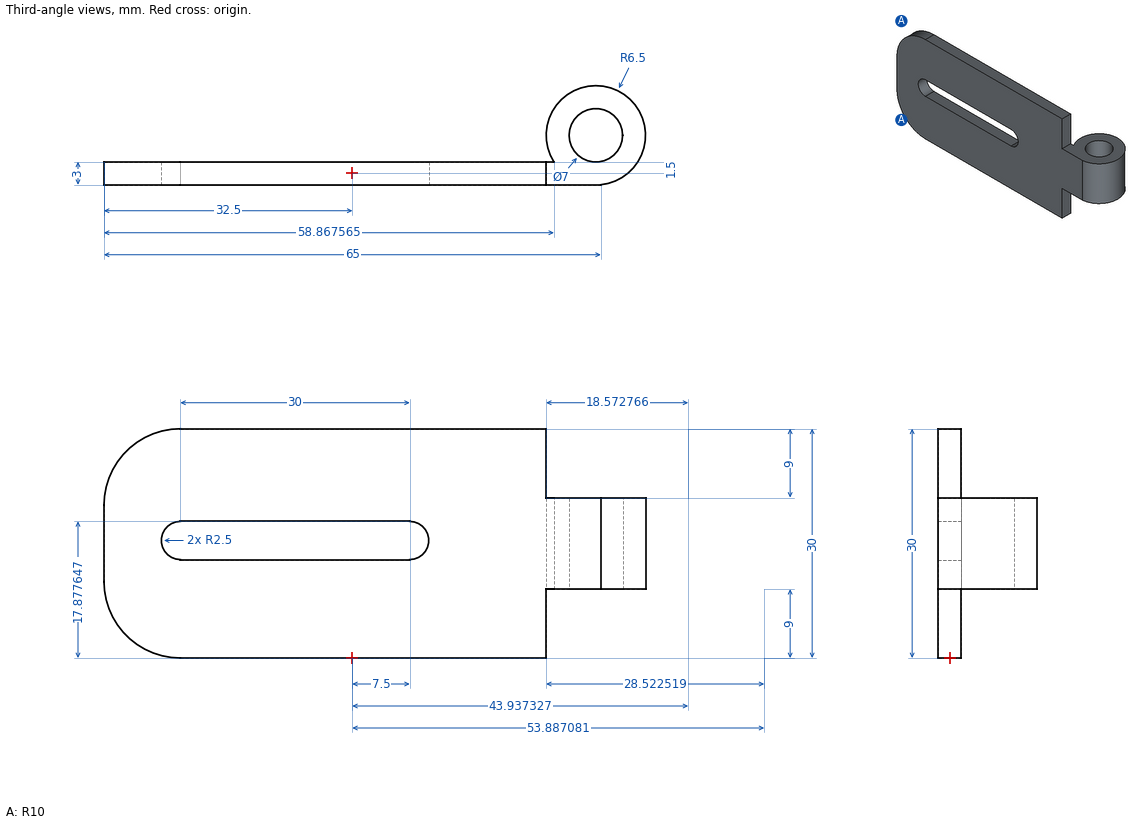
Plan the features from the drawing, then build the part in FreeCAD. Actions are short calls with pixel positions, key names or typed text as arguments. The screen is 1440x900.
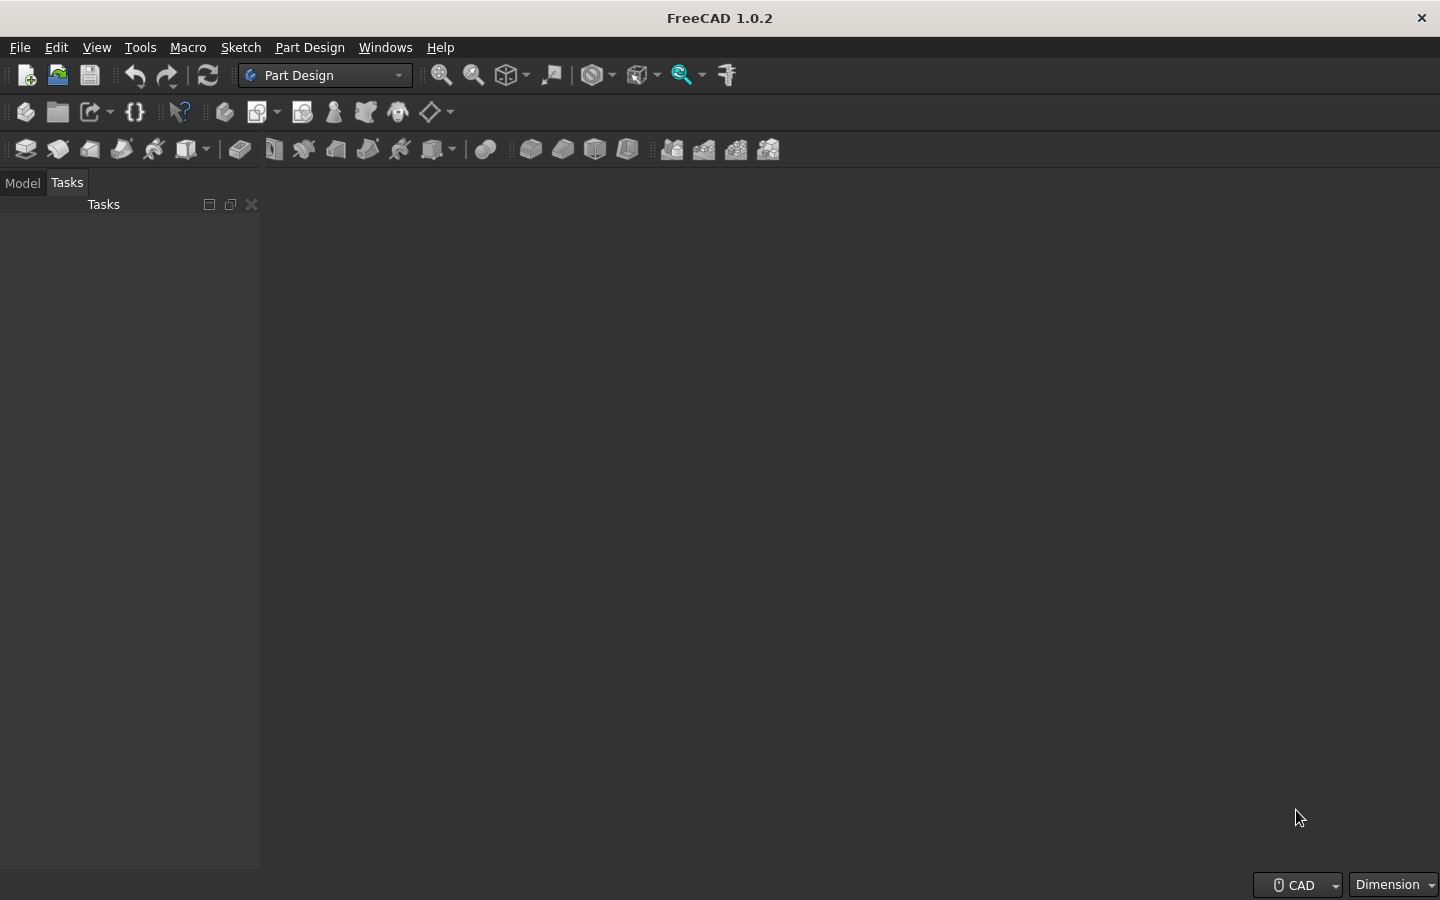
click(286, 112)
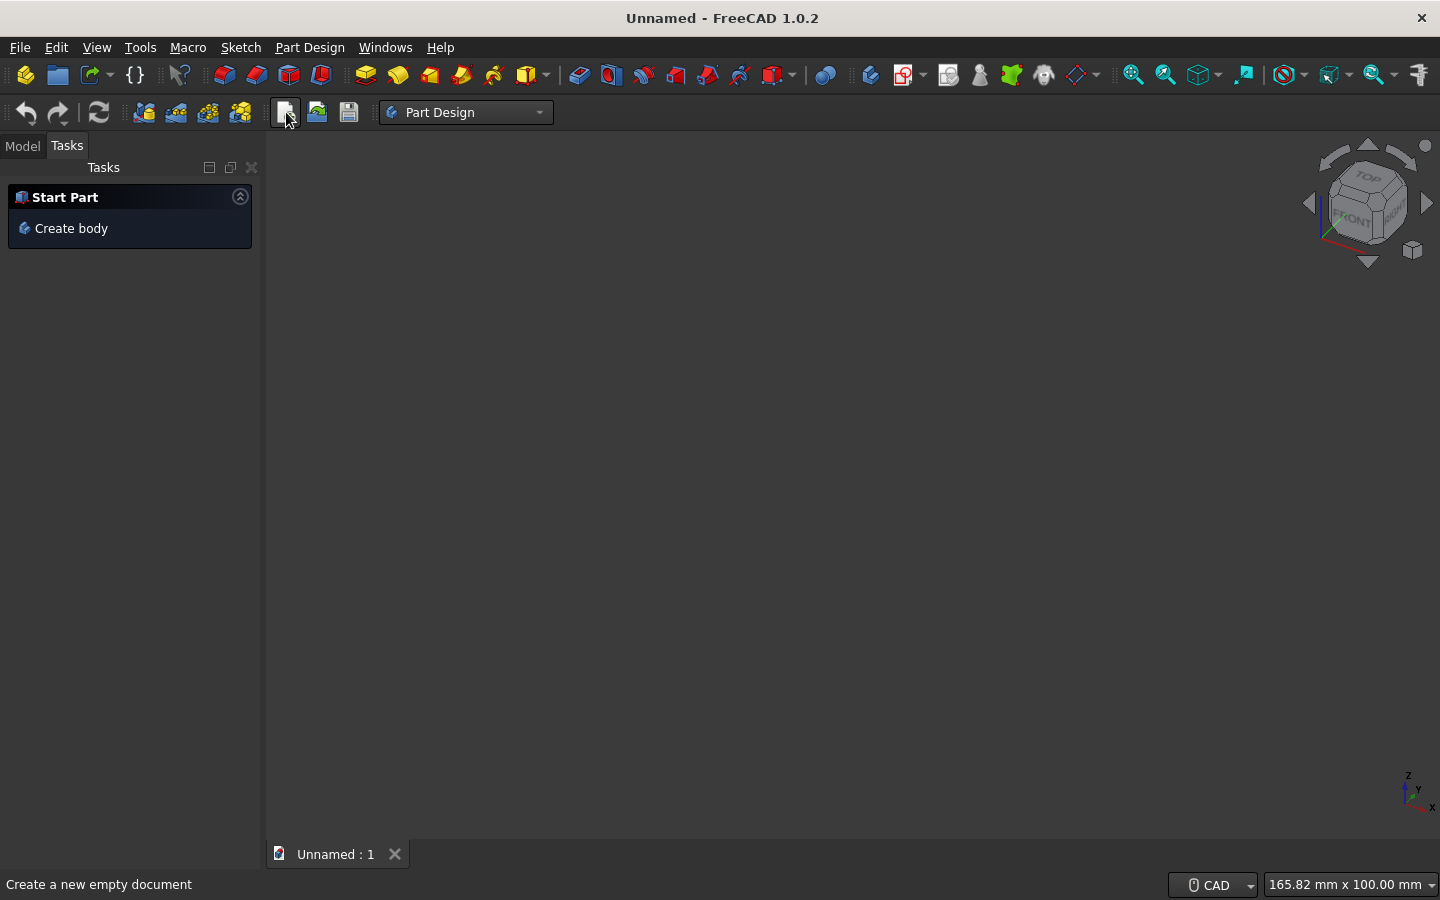
click(904, 76)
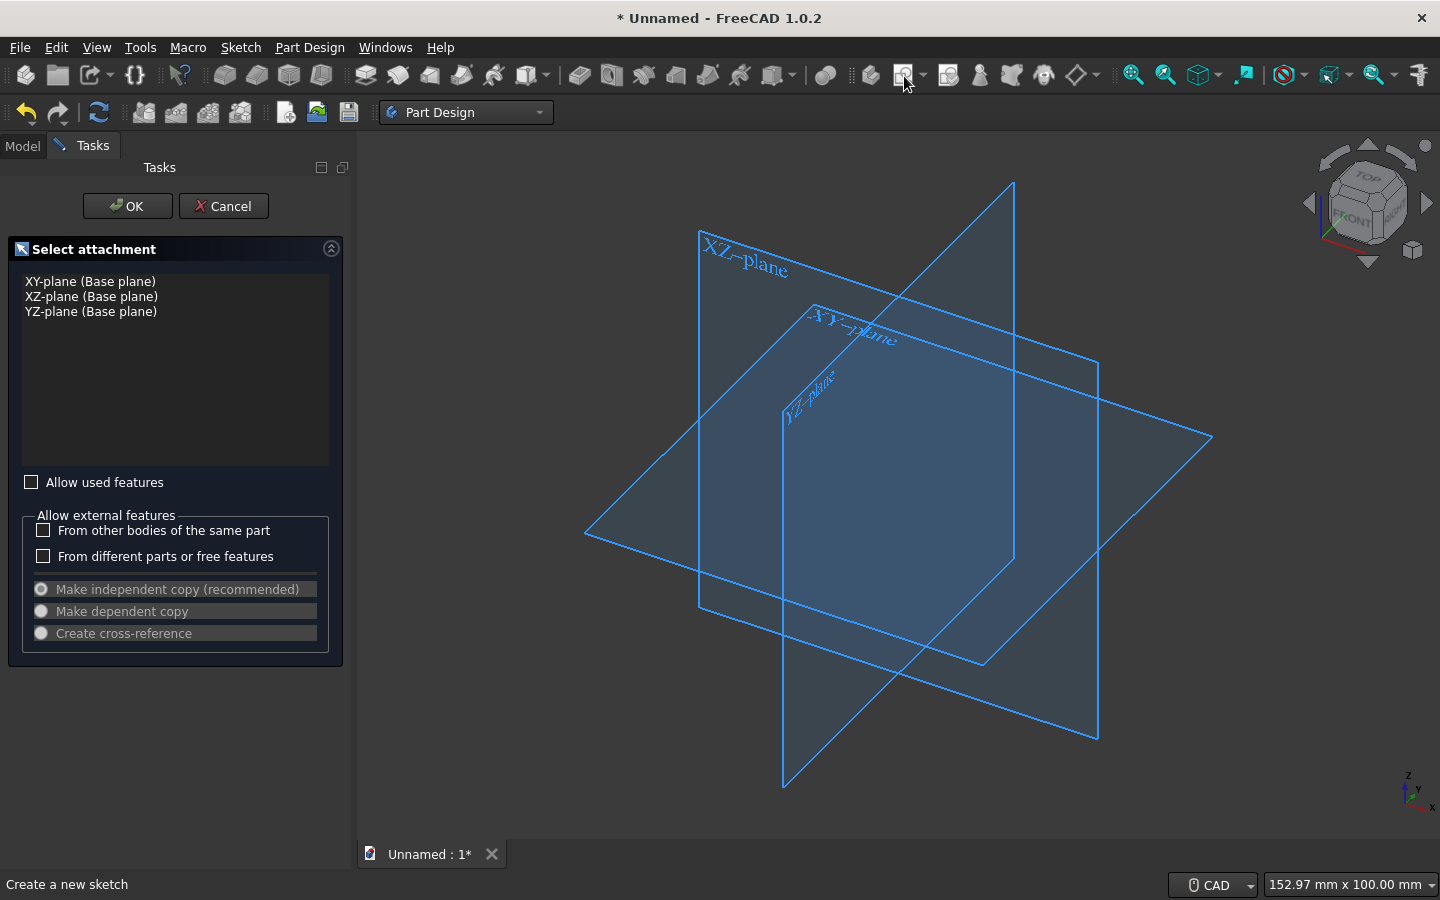
click(82, 282)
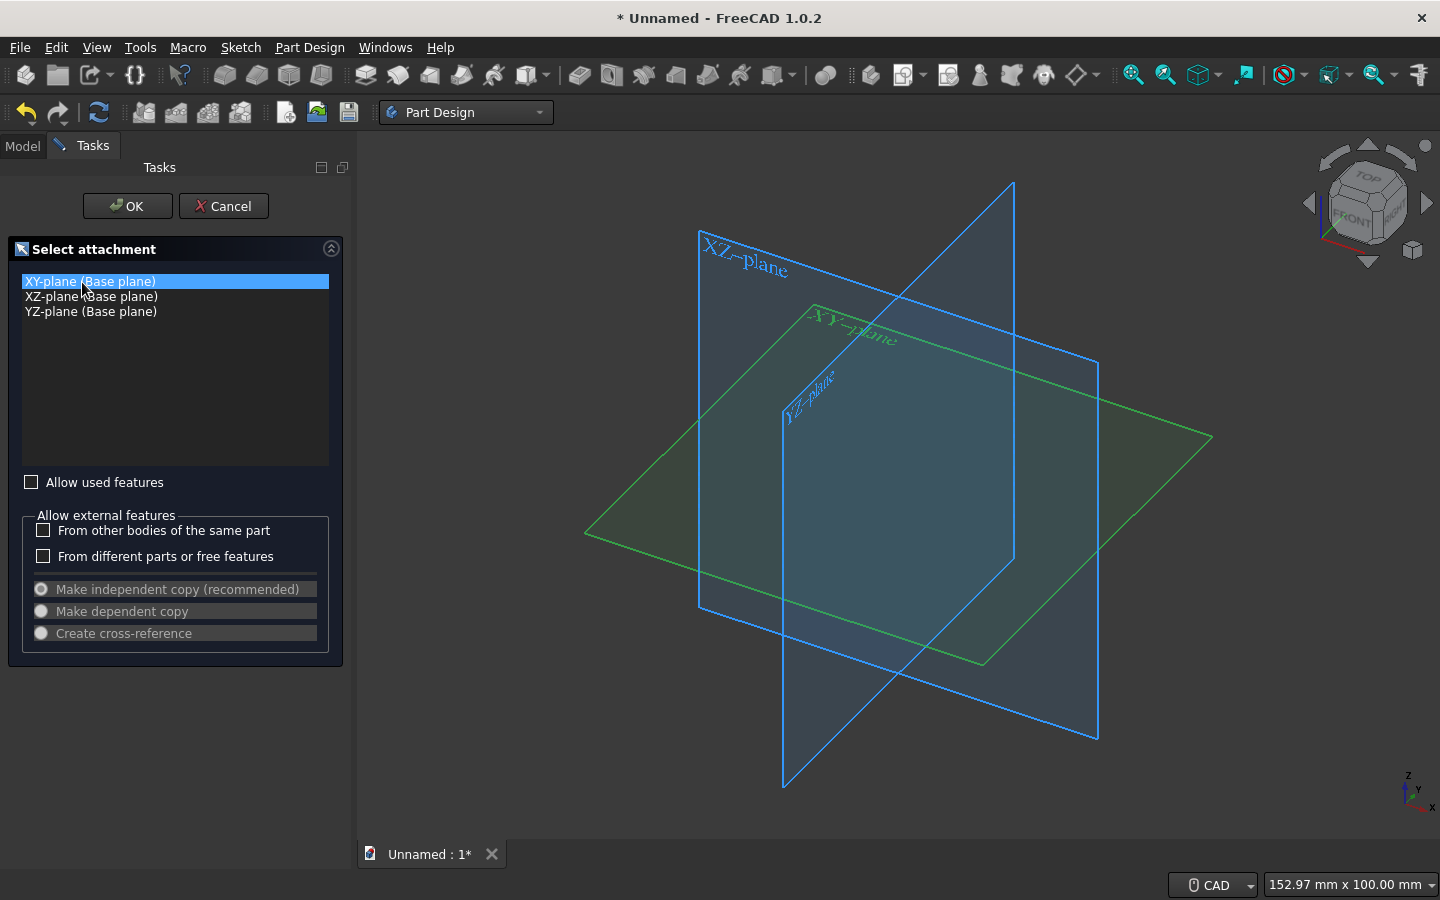
click(128, 206)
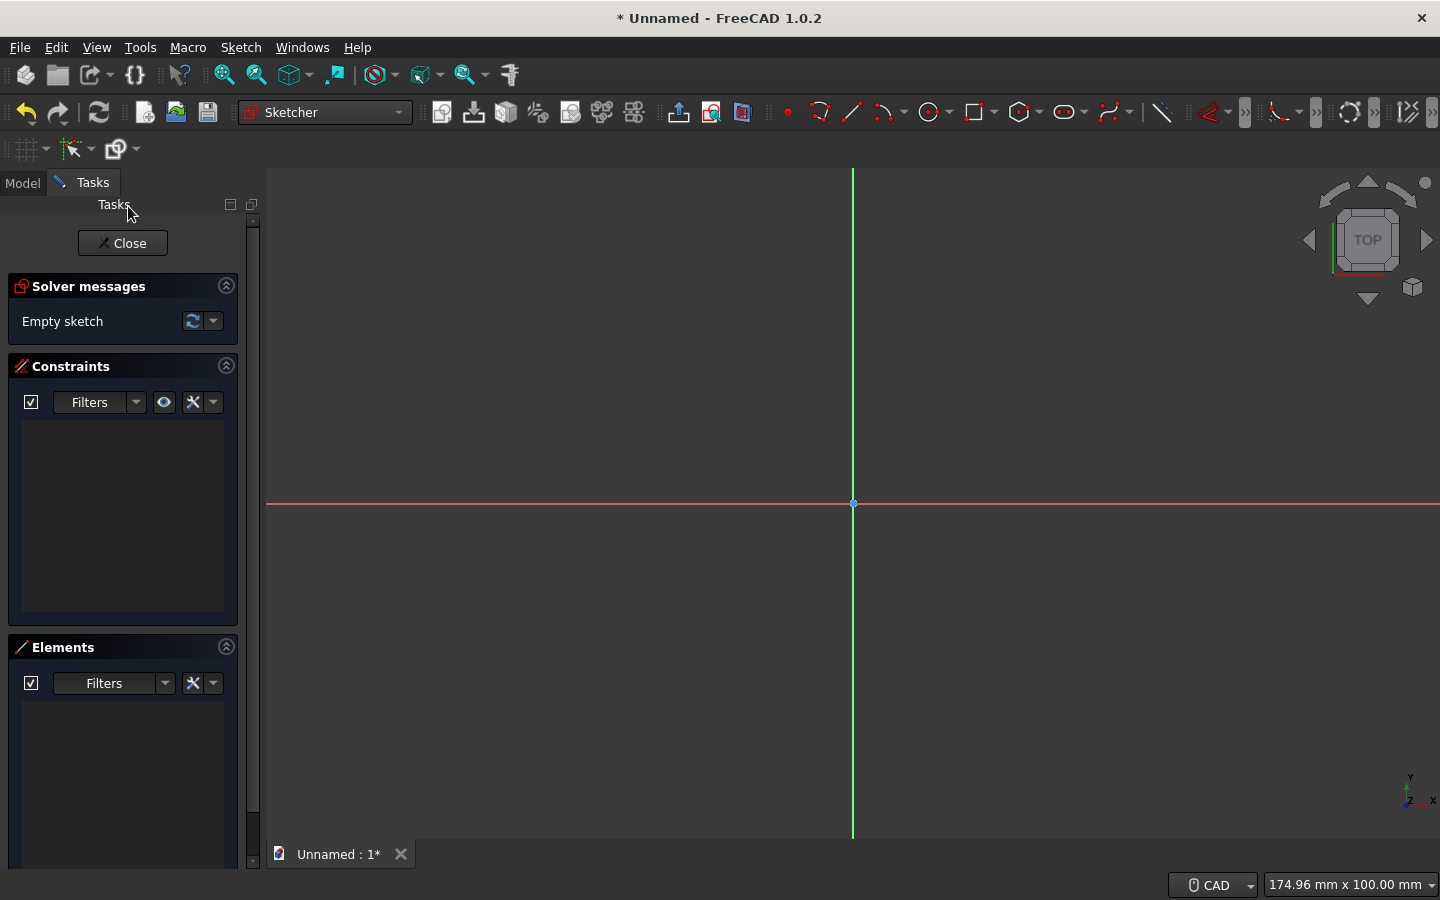
scroll(1021, 409, up, 2)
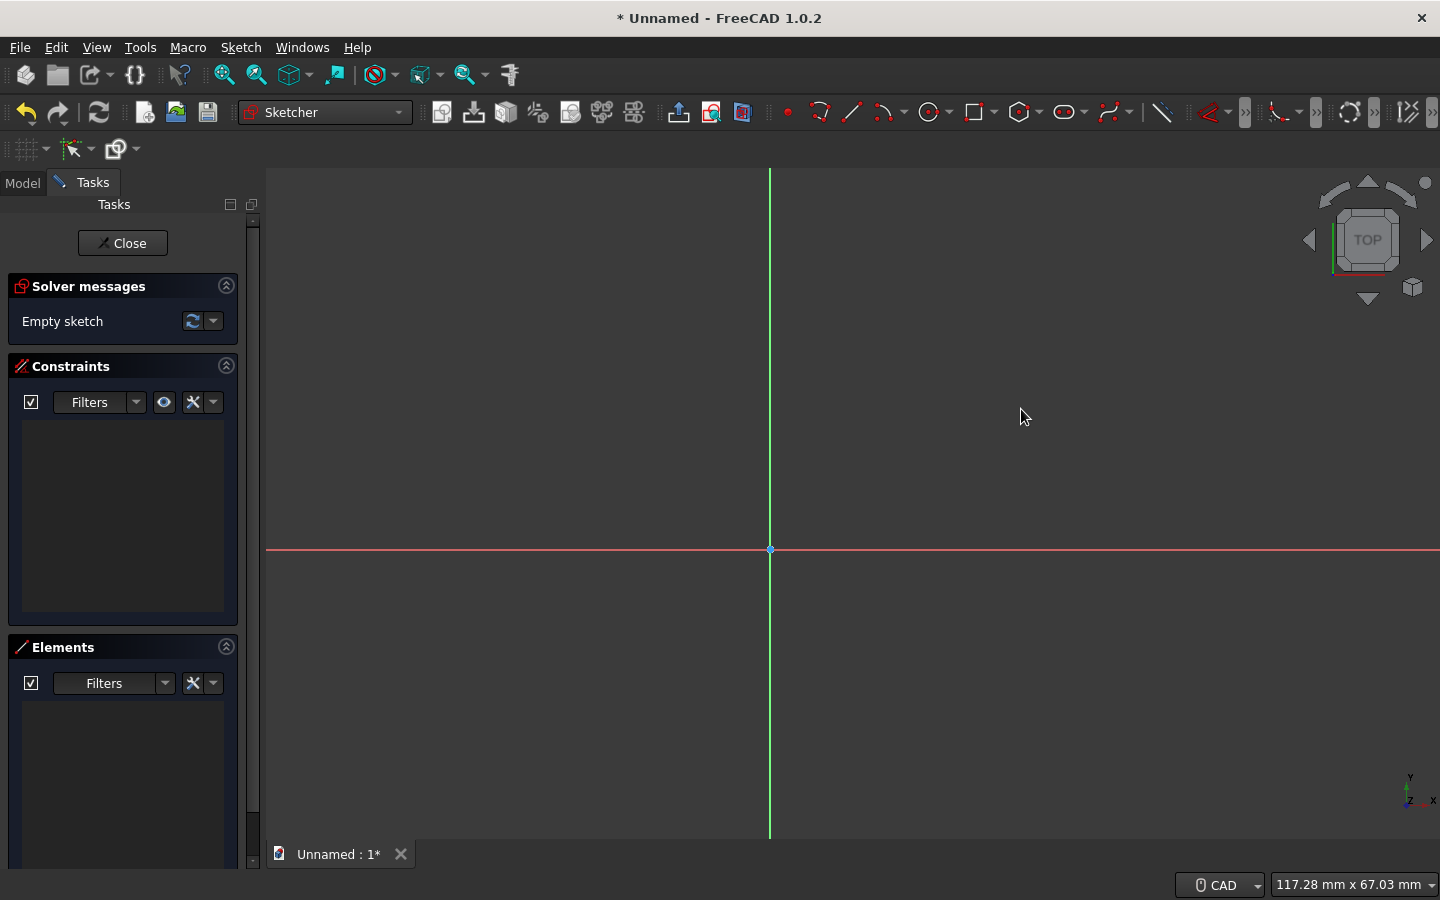
click(820, 112)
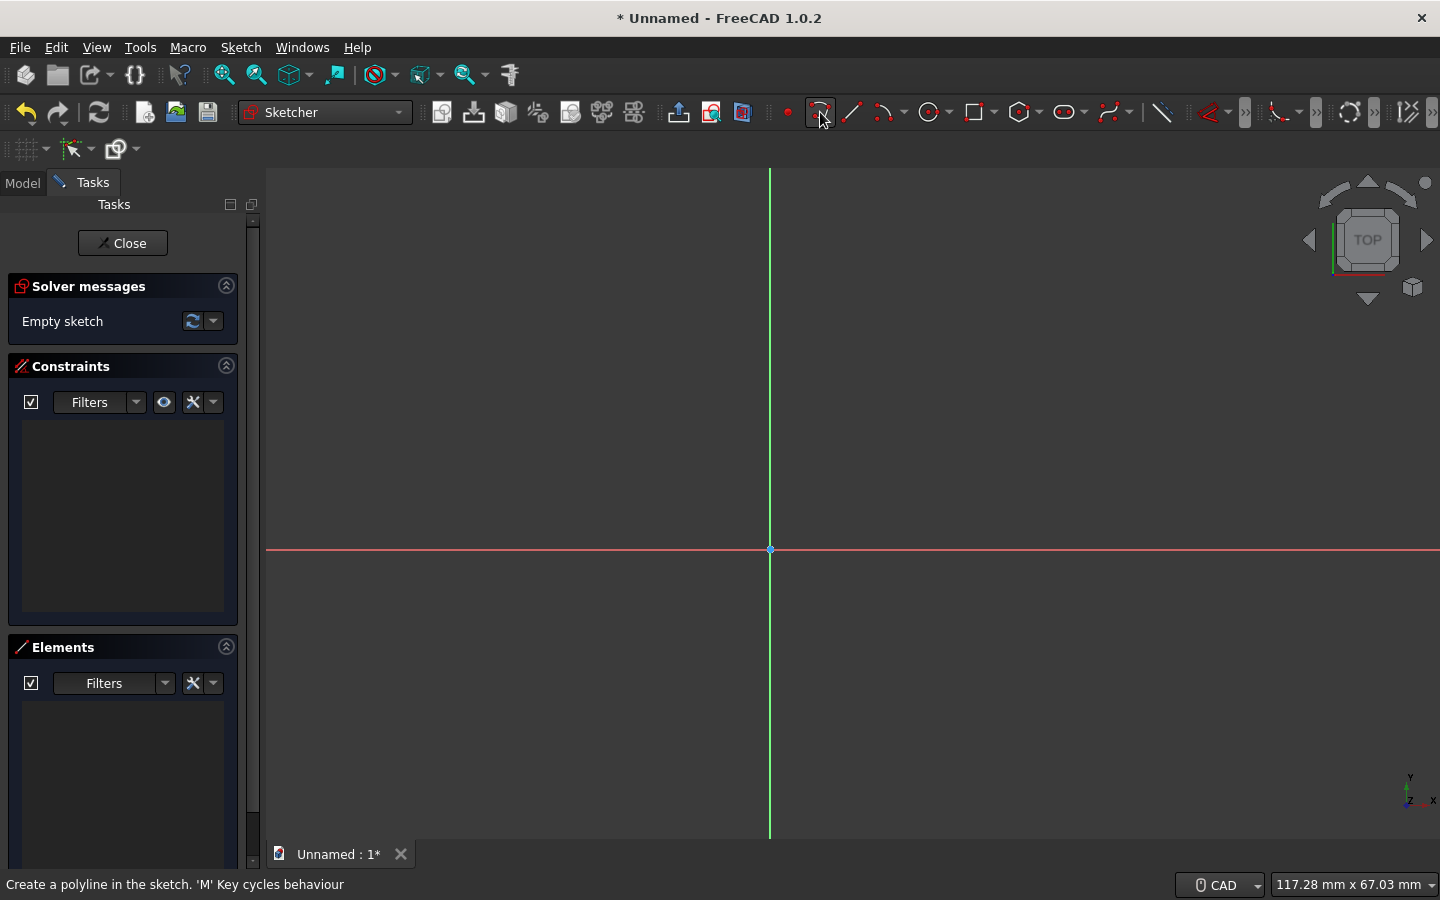
click(1034, 535)
click(445, 535)
click(445, 565)
click(1095, 565)
right_click(1095, 565)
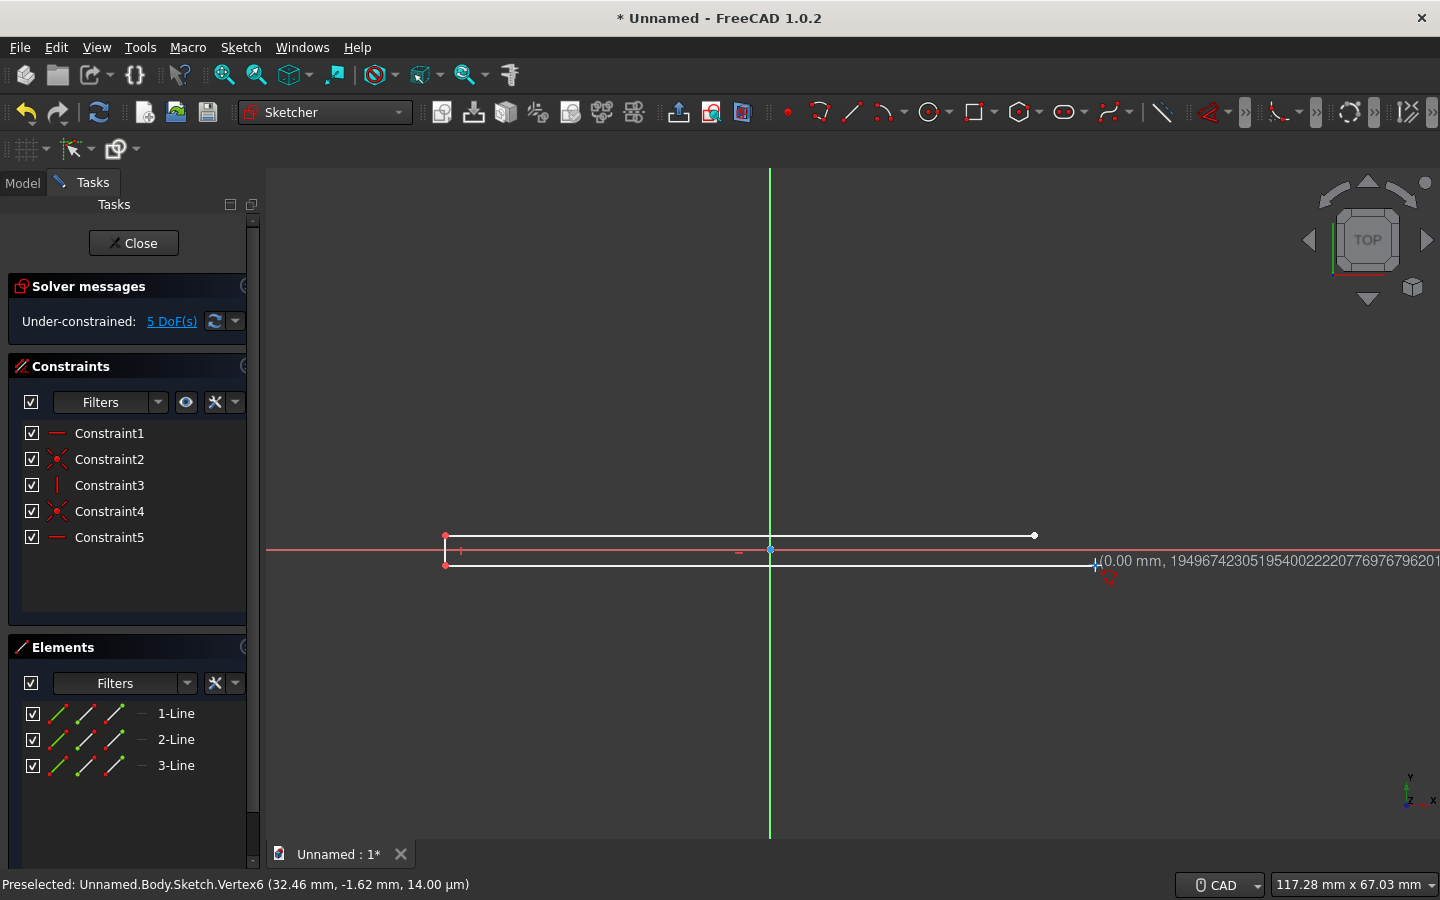
key(g)
key(3)
key(a)